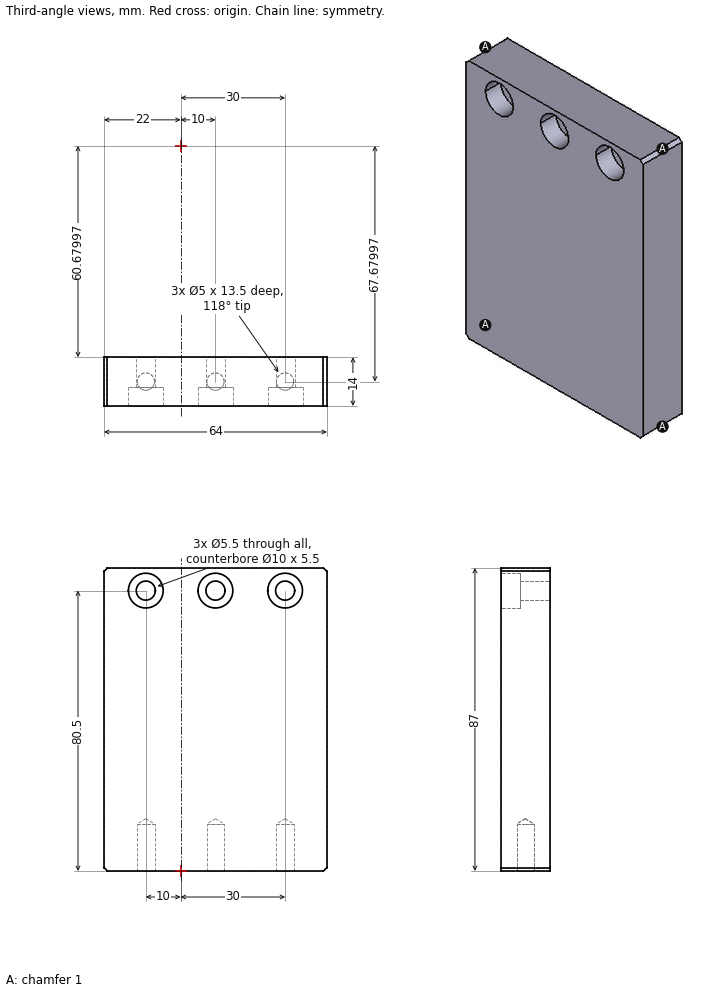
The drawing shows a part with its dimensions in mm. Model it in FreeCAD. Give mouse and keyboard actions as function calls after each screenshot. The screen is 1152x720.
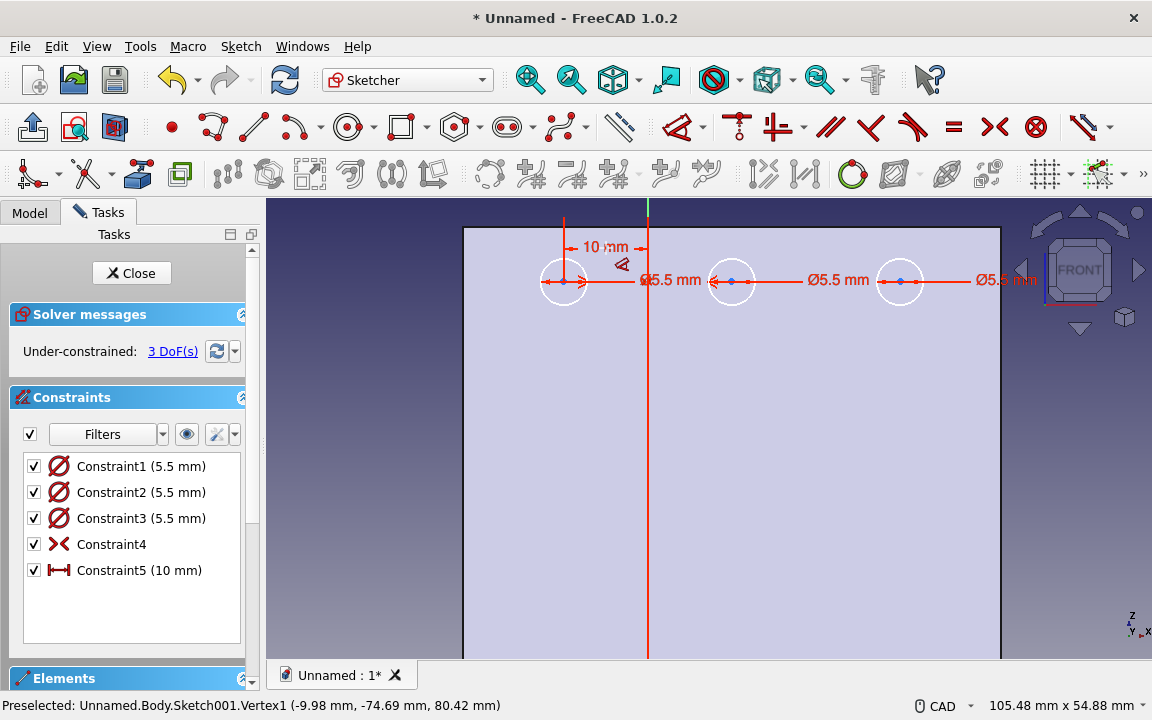
click(900, 282)
click(774, 248)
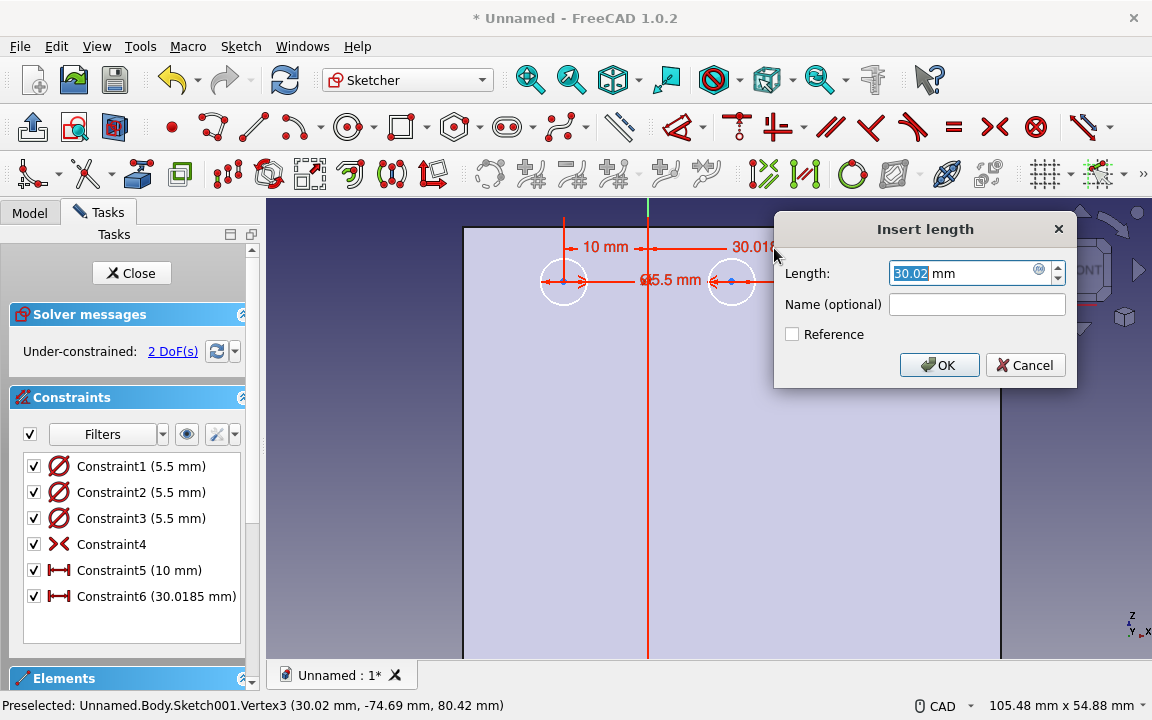
text(30)
key(Return)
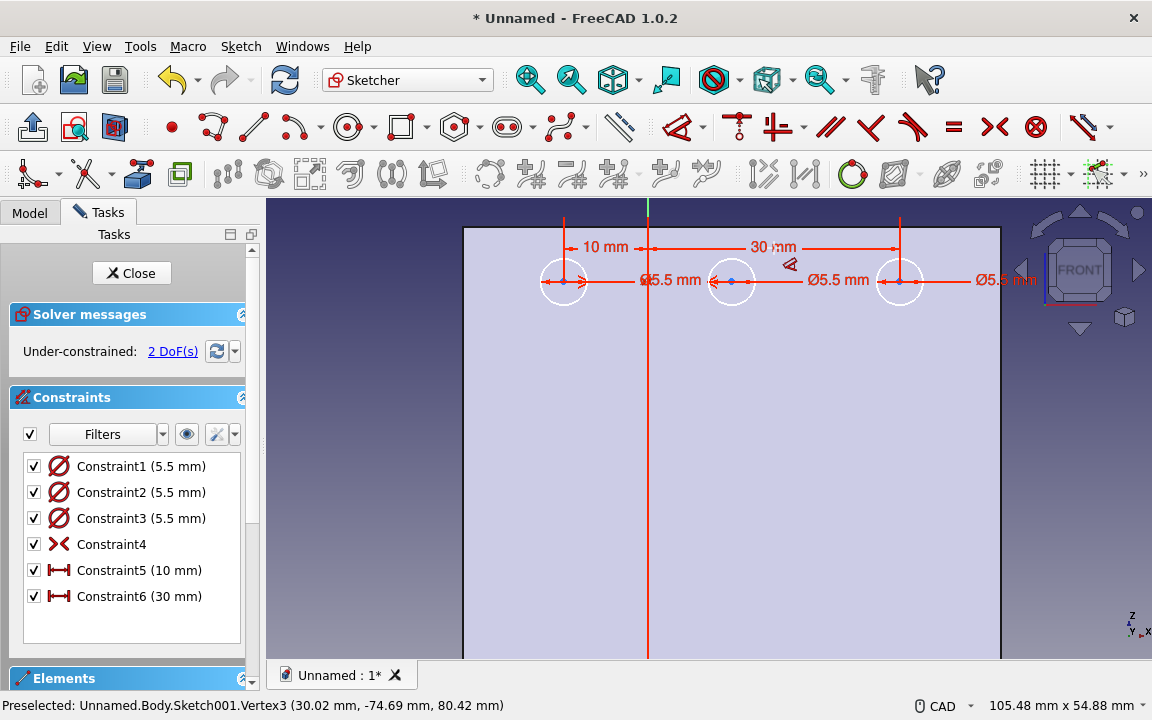
click(564, 282)
click(530, 456)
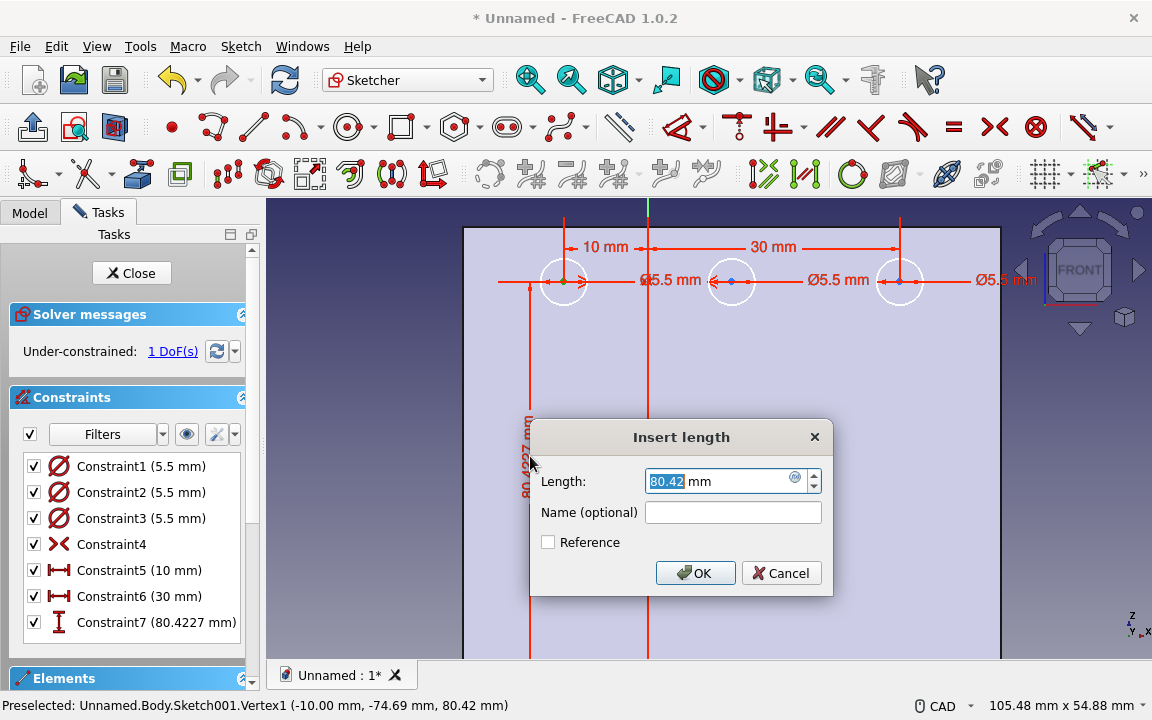
text(80.5)
key(Return)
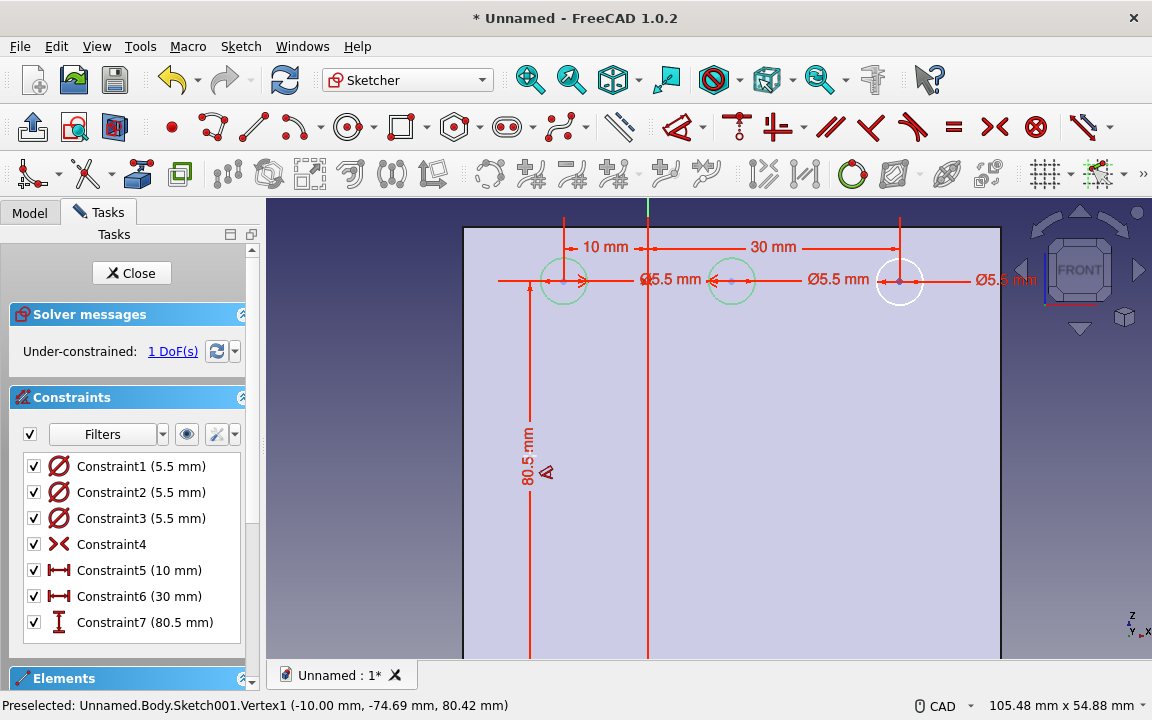
click(900, 282)
click(934, 456)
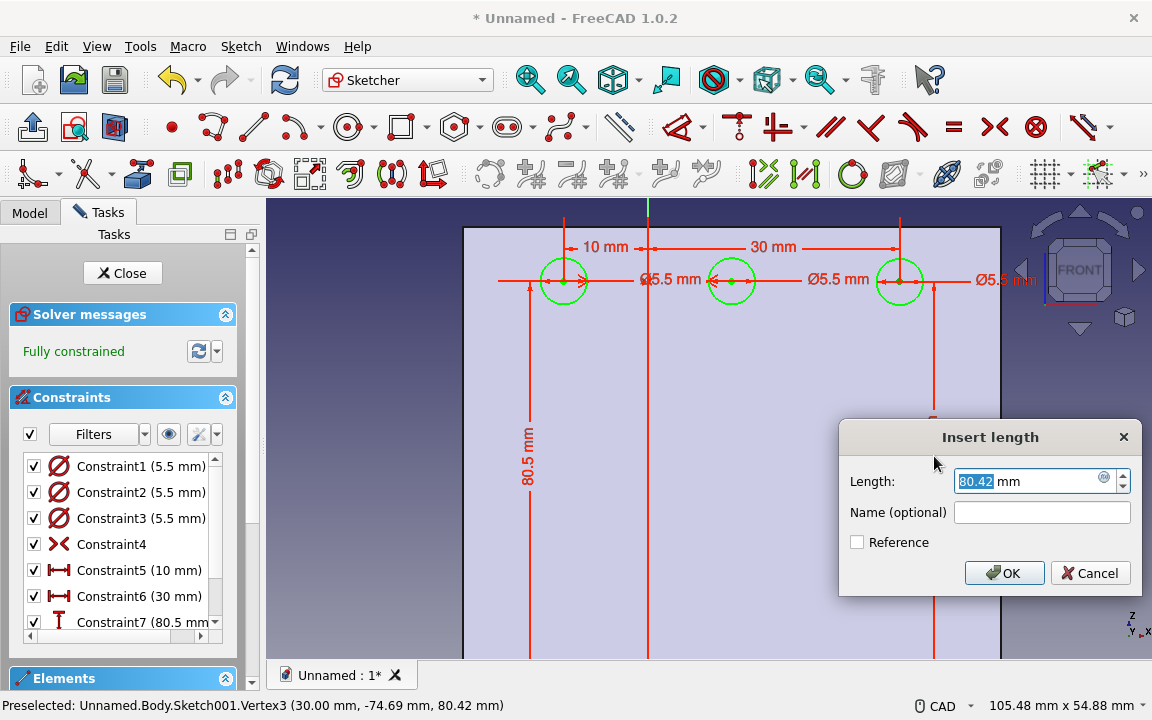
text(80.5)
key(Return)
key(Escape)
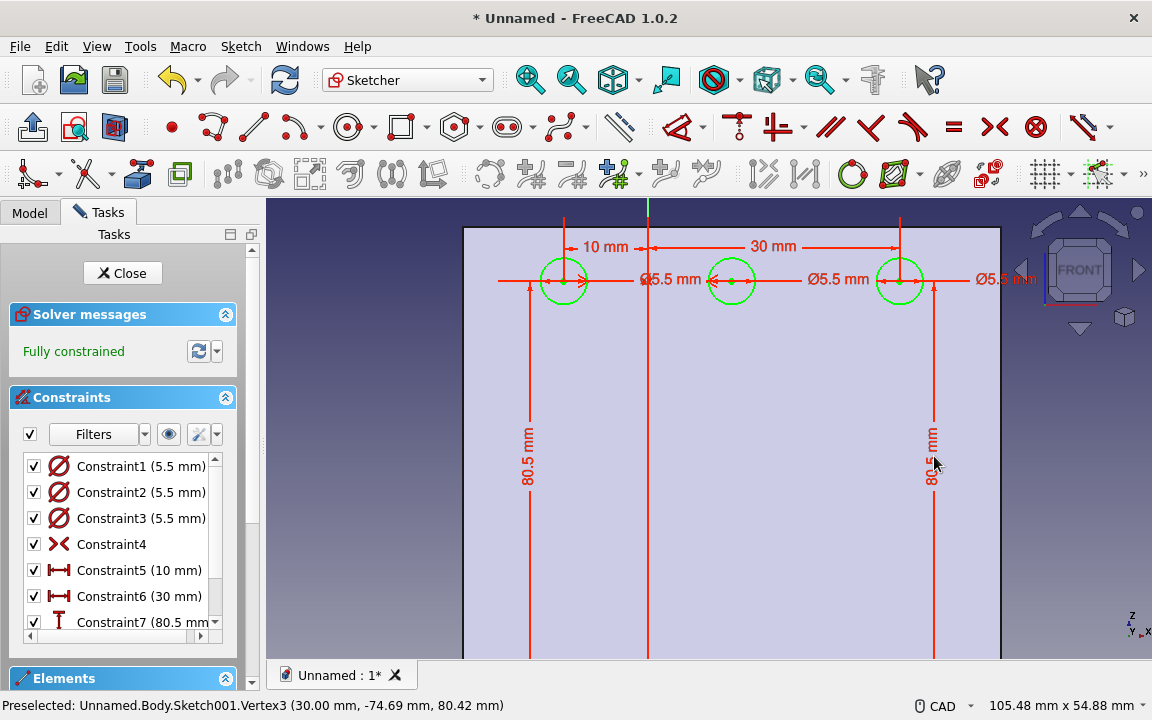
click(123, 273)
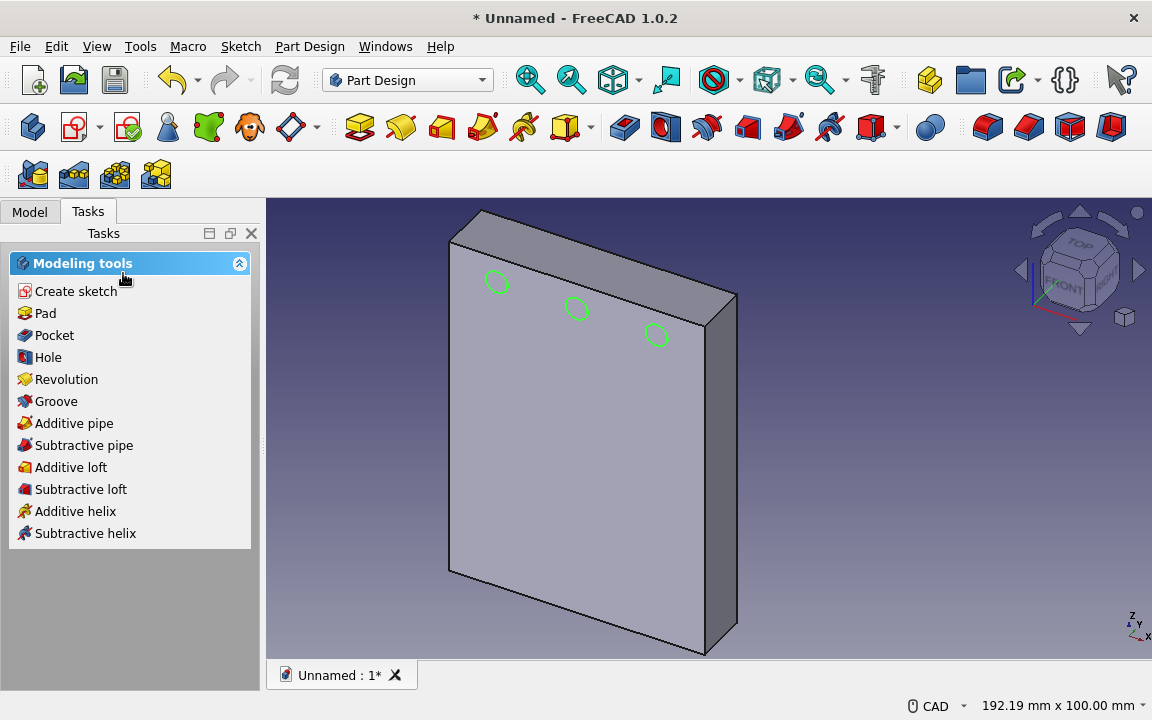
click(666, 128)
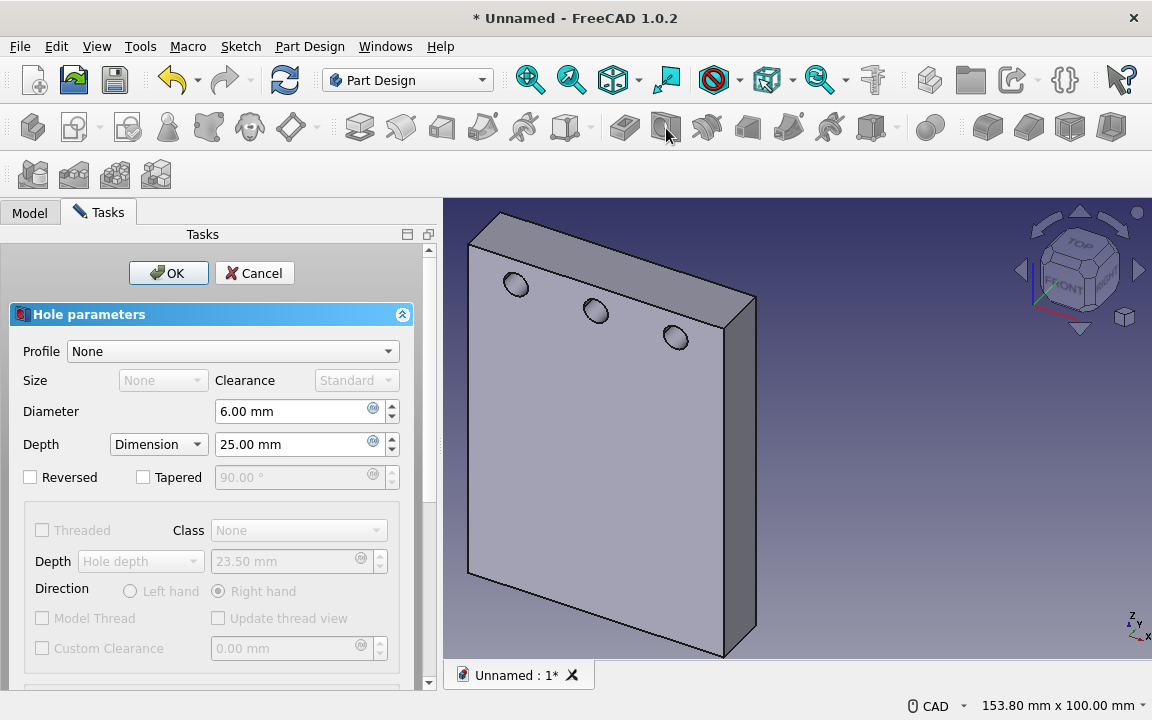
triple_click(300, 412)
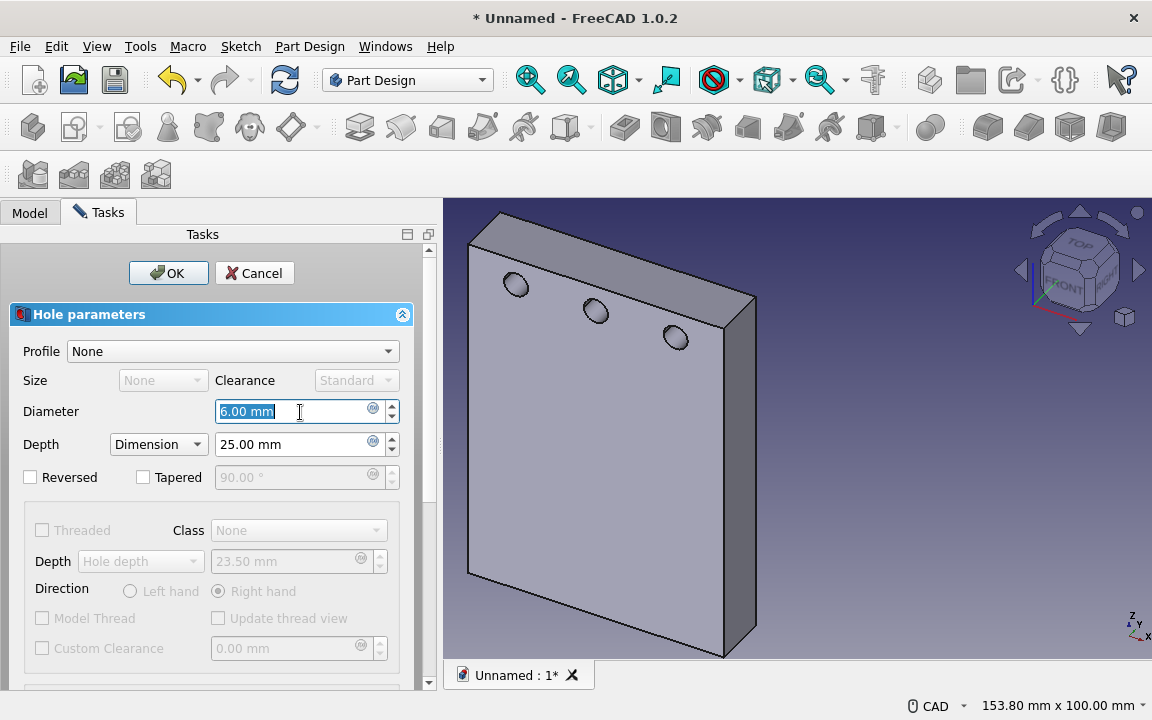
text(5.5)
key(Tab)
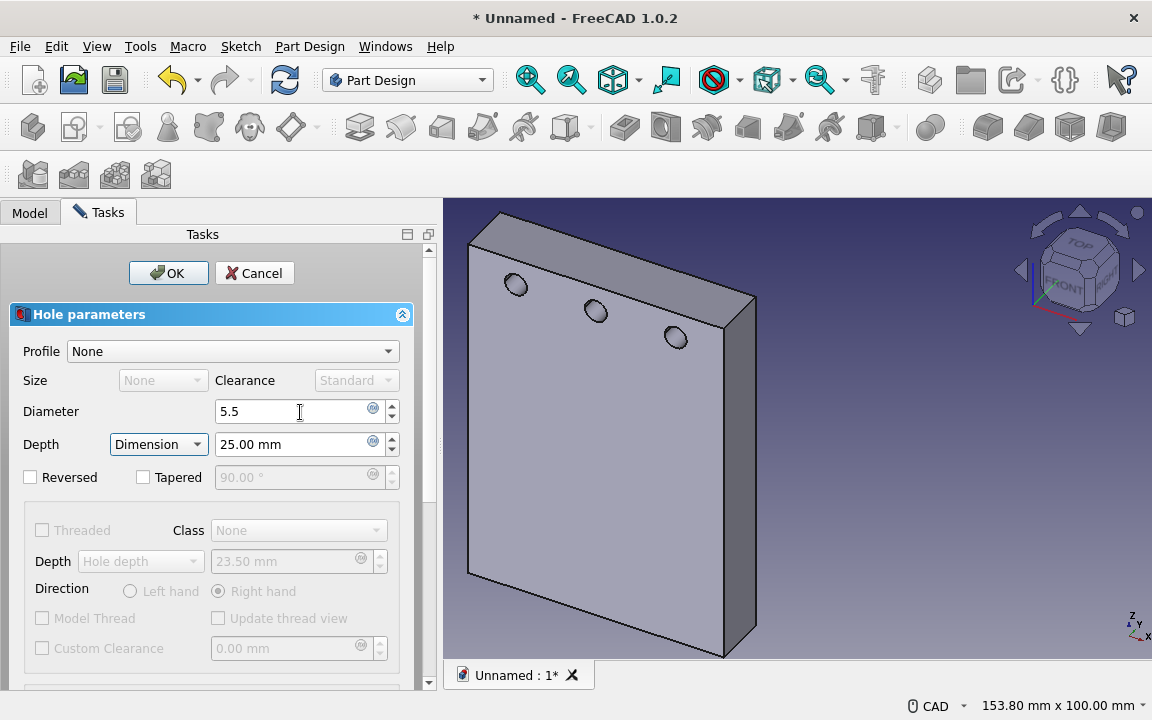
click(160, 444)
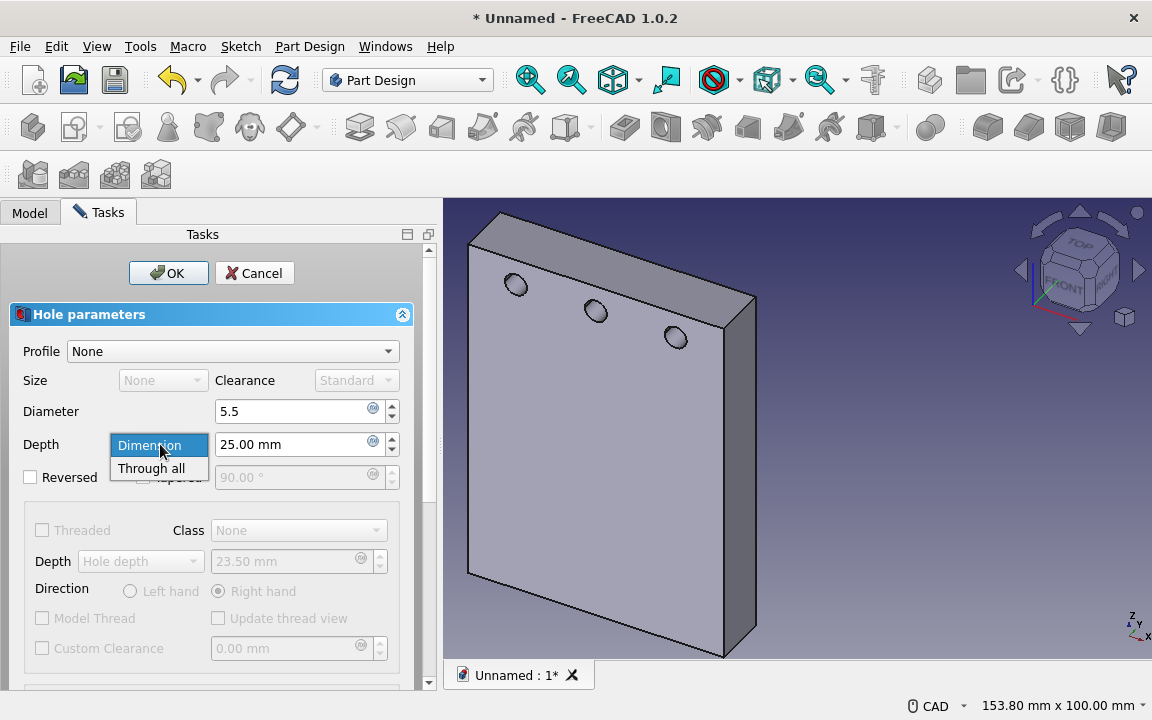
click(158, 468)